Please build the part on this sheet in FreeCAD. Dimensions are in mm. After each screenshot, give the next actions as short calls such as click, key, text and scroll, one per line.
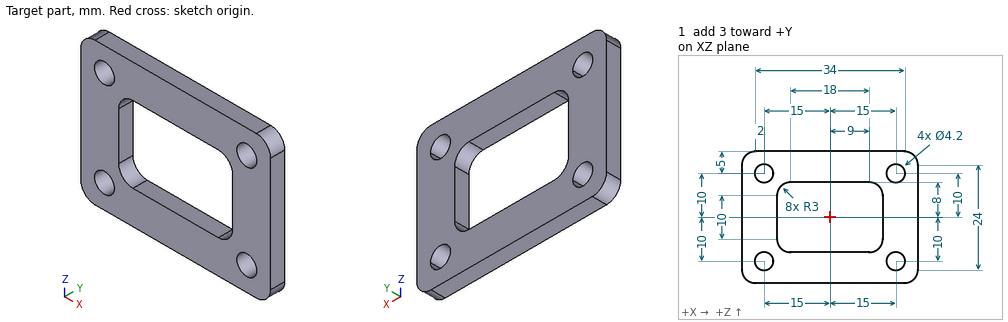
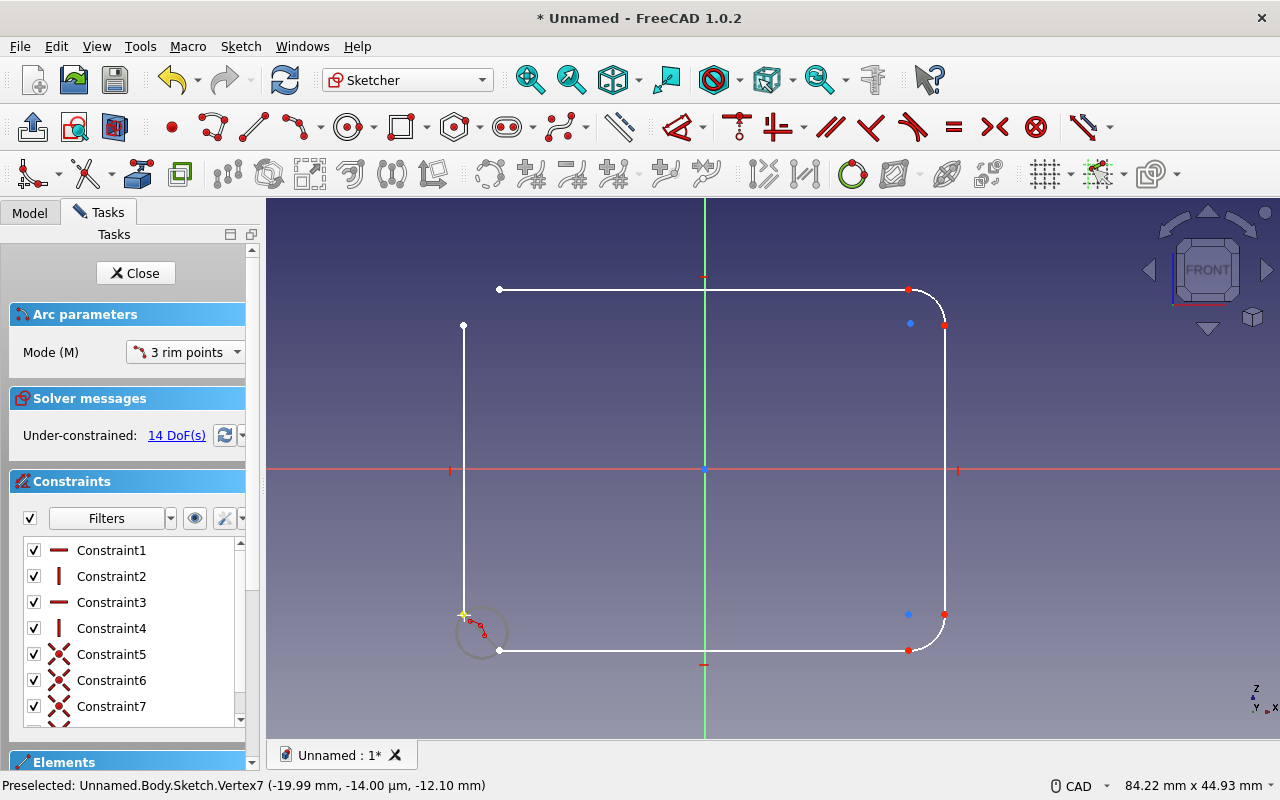
scroll(474, 639, up, 3)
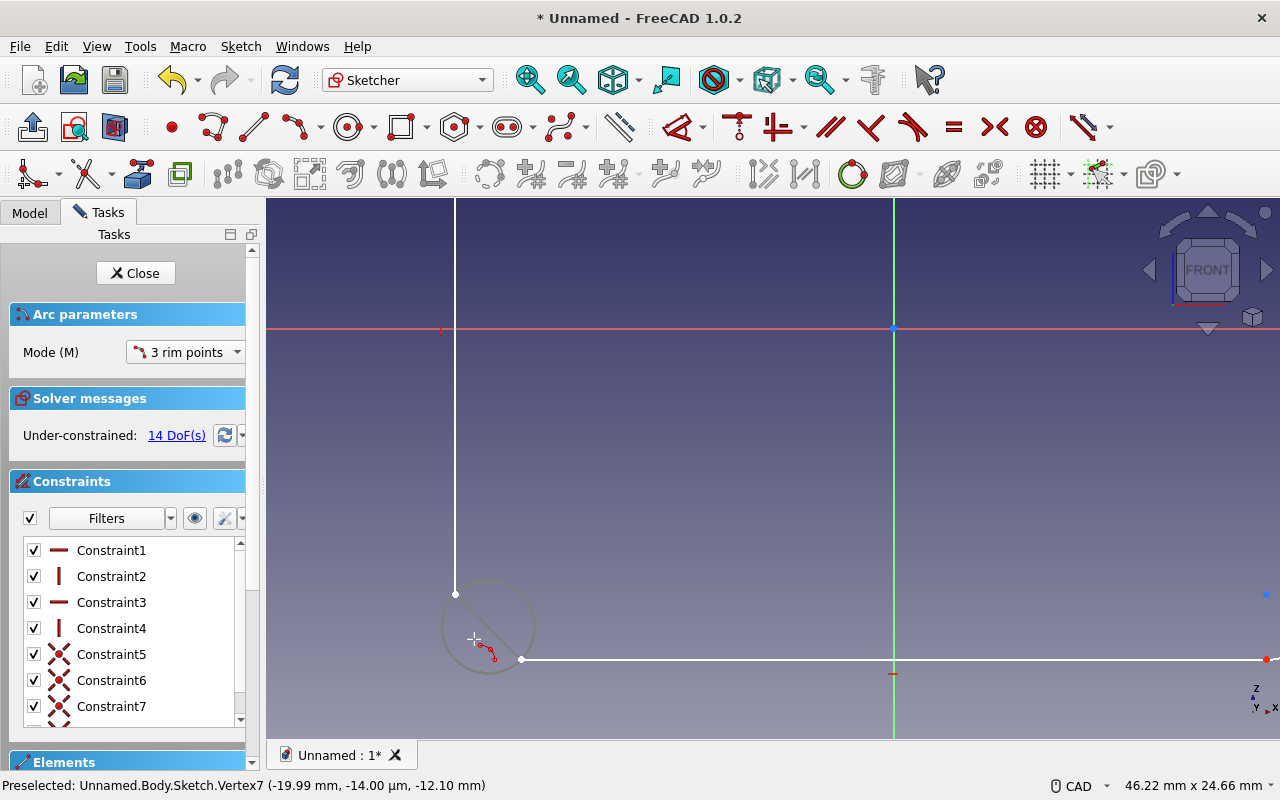
click(475, 639)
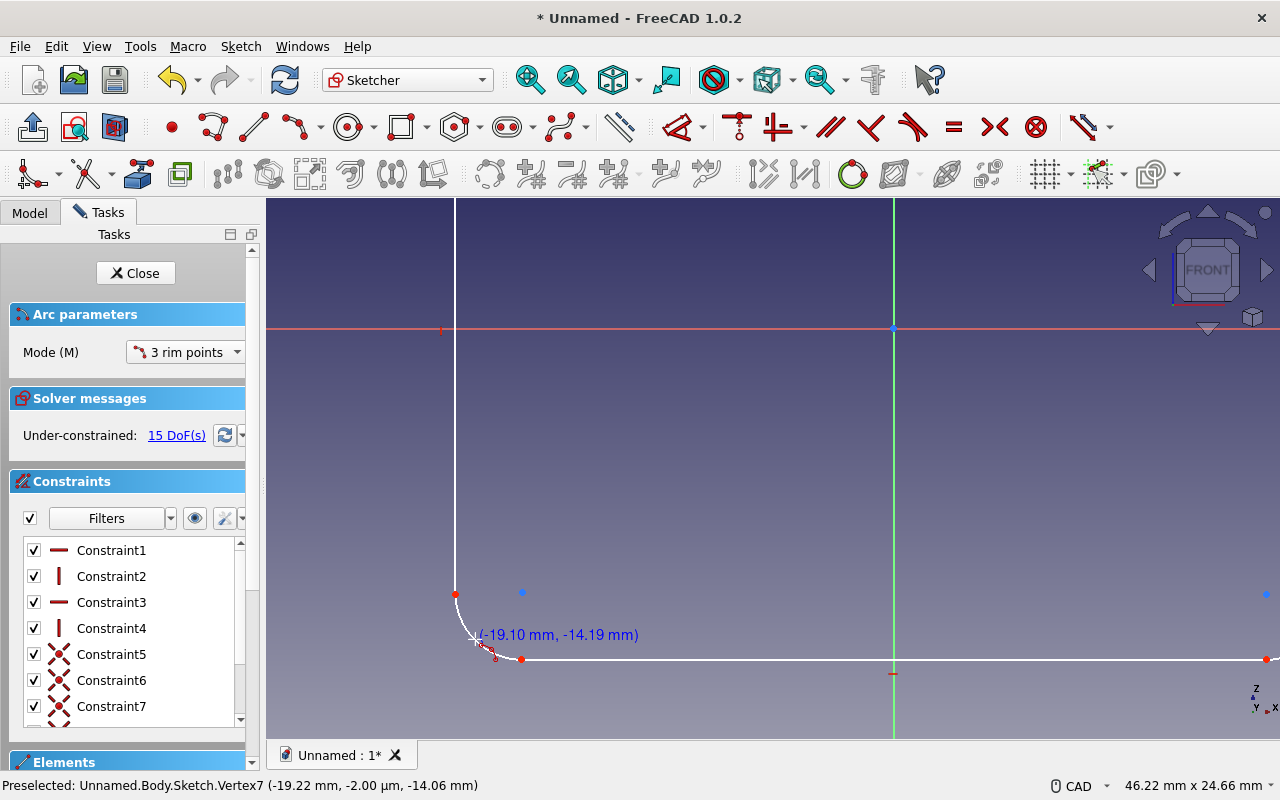
scroll(474, 639, down, 3)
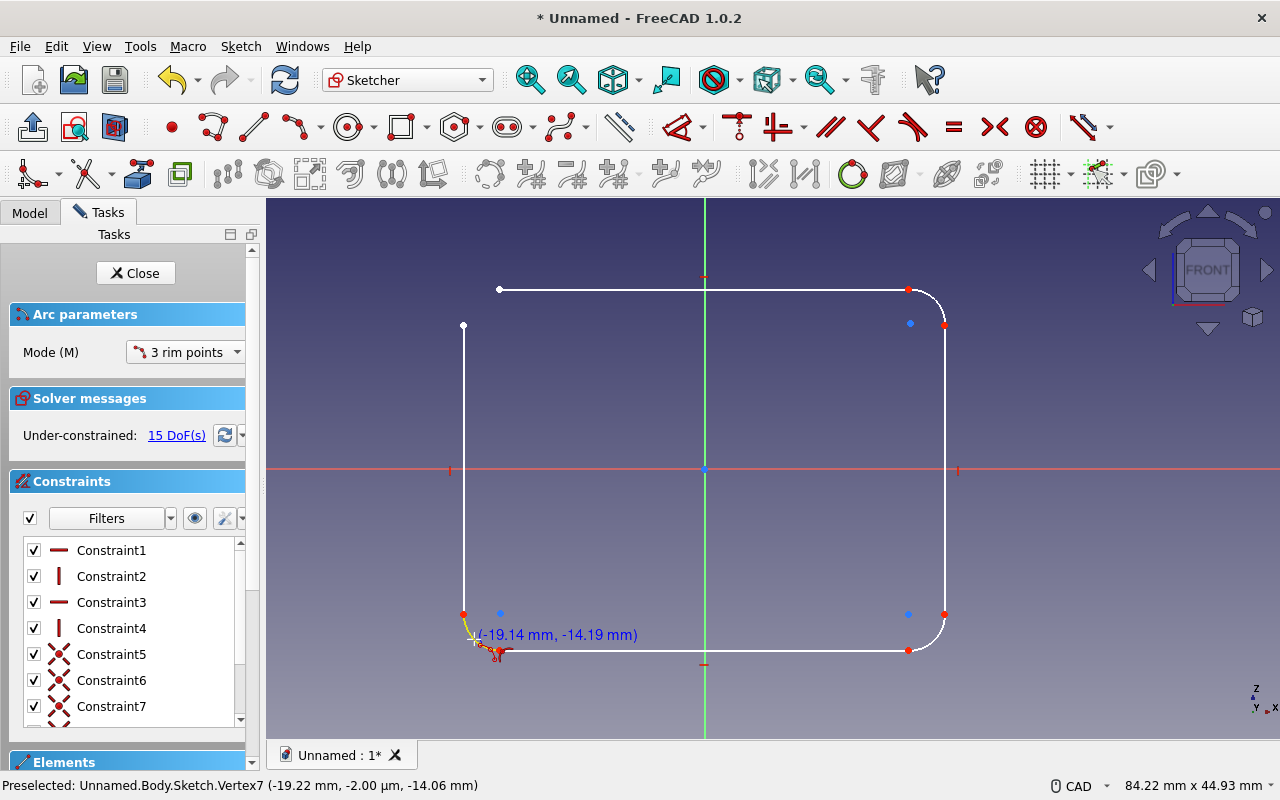
click(464, 326)
click(500, 290)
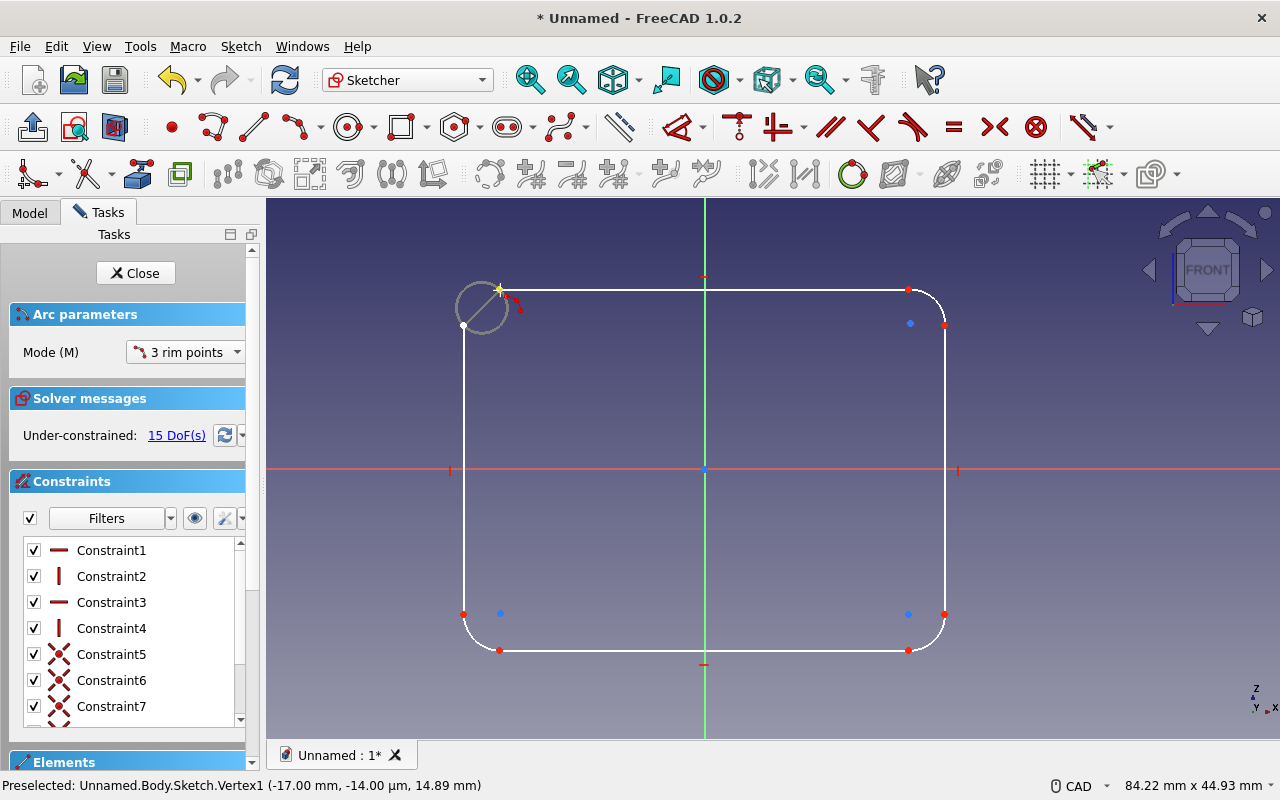
scroll(474, 299, up, 3)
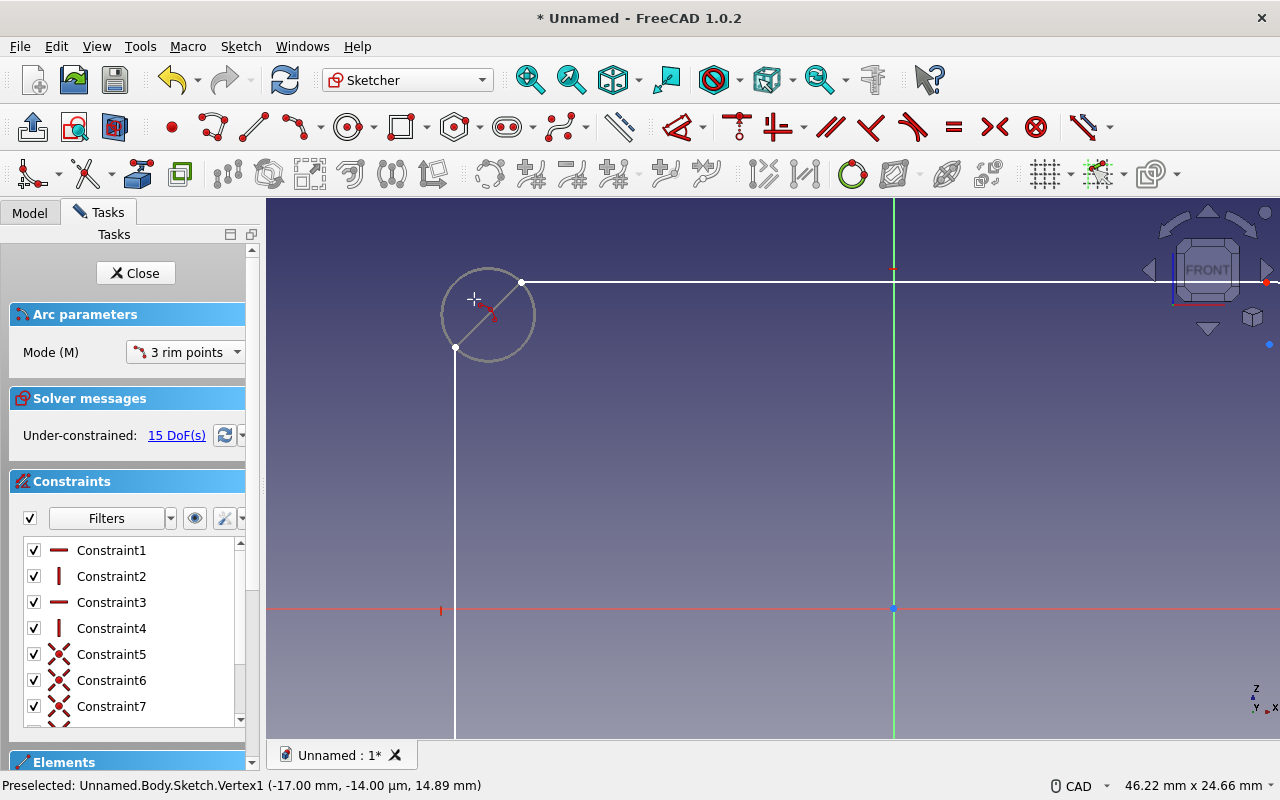
click(475, 299)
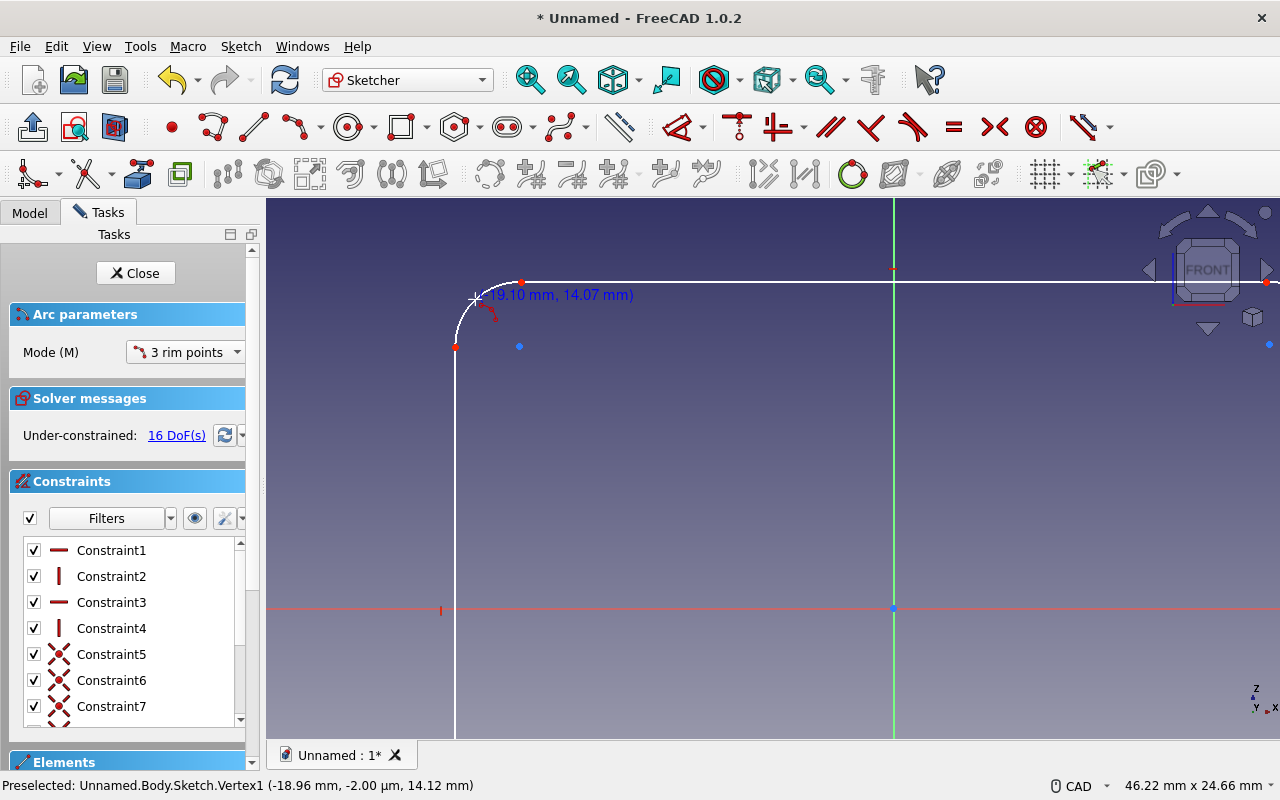
key(g)
key(l)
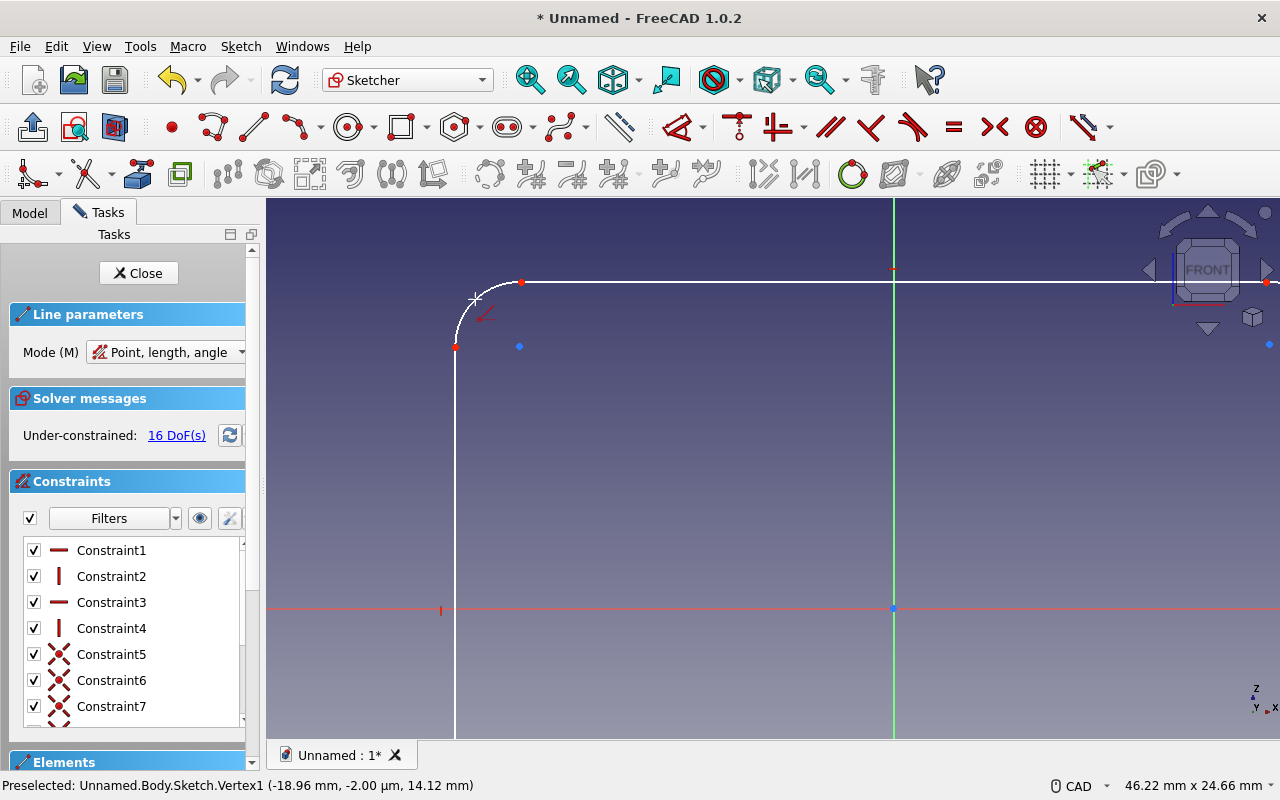
click(1091, 433)
click(697, 433)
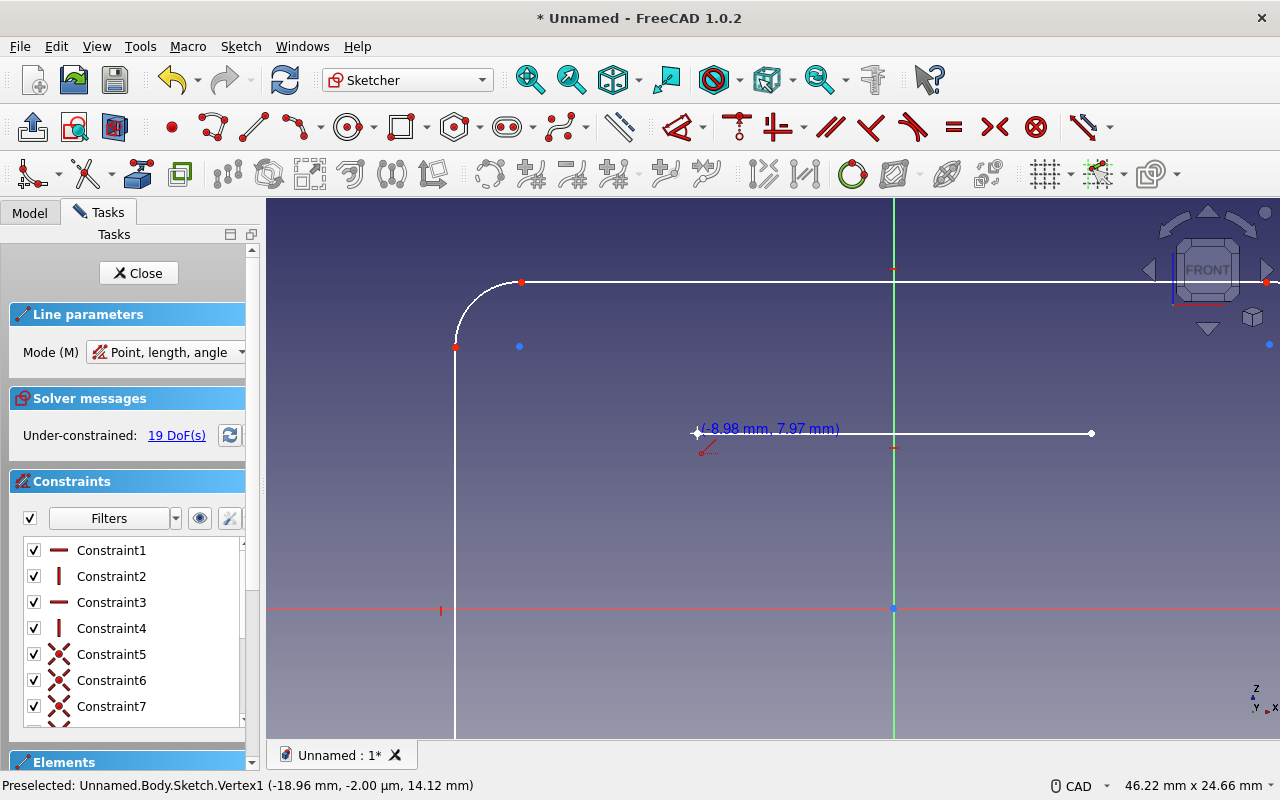
click(631, 499)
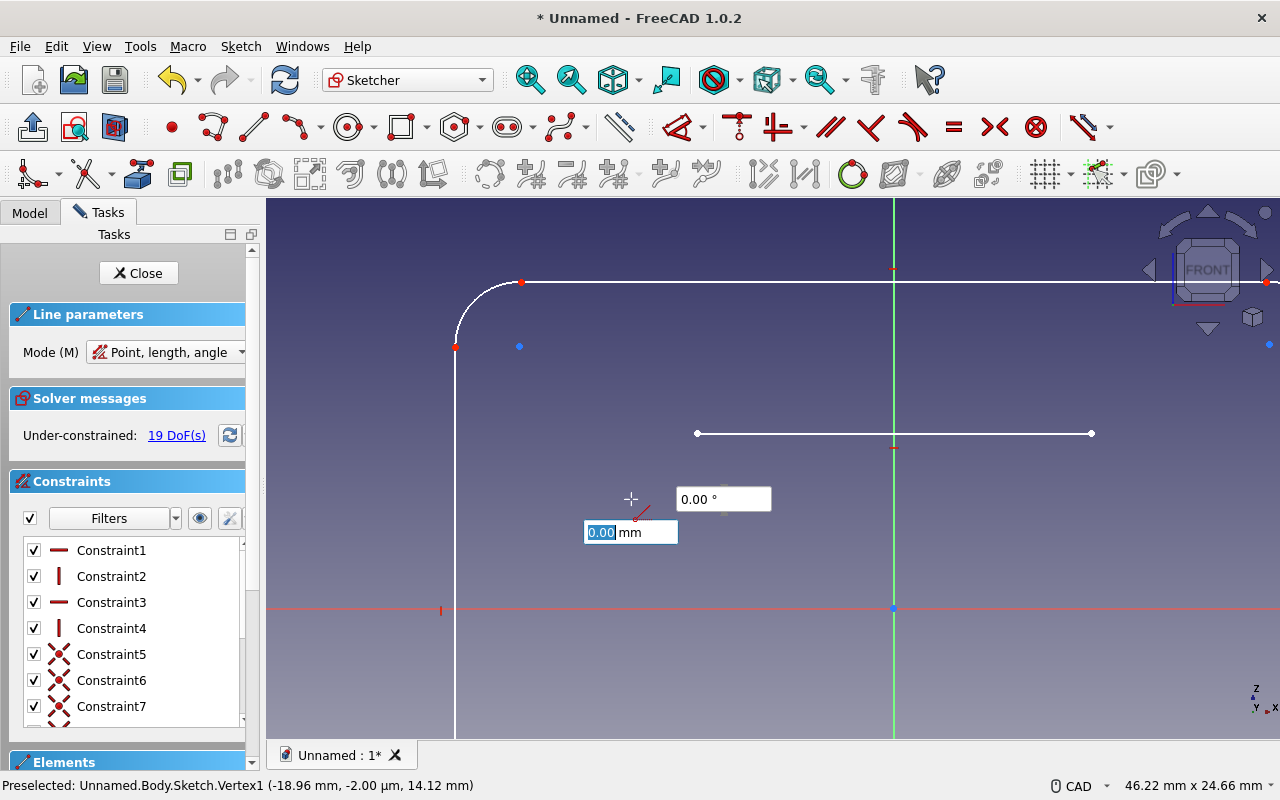
scroll(474, 298, down, 3)